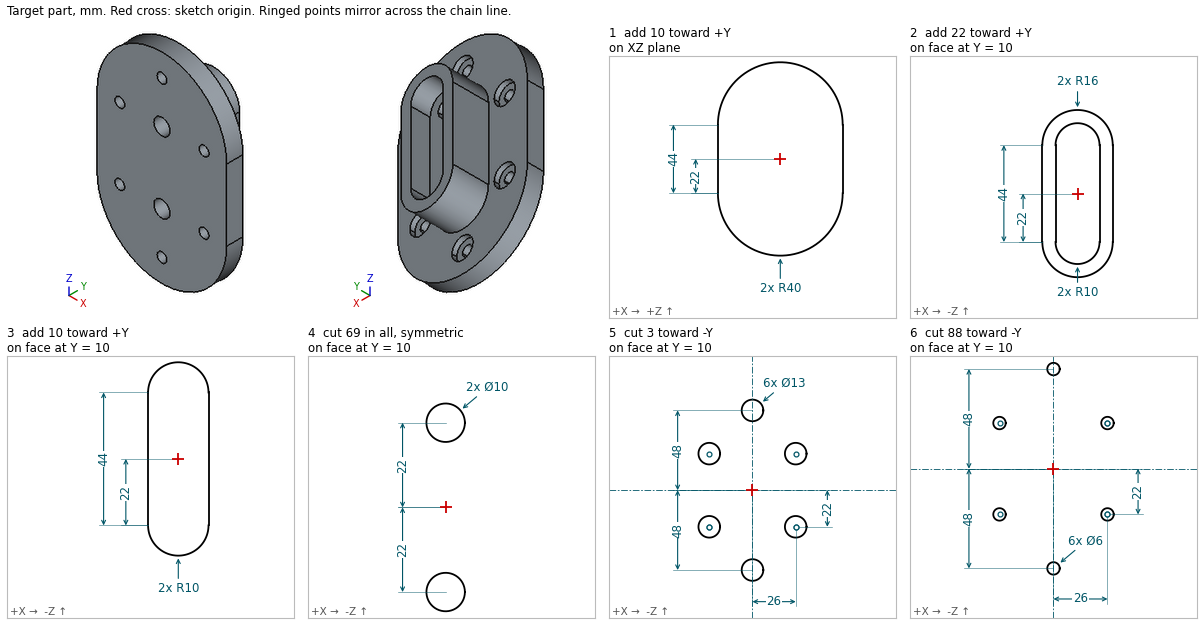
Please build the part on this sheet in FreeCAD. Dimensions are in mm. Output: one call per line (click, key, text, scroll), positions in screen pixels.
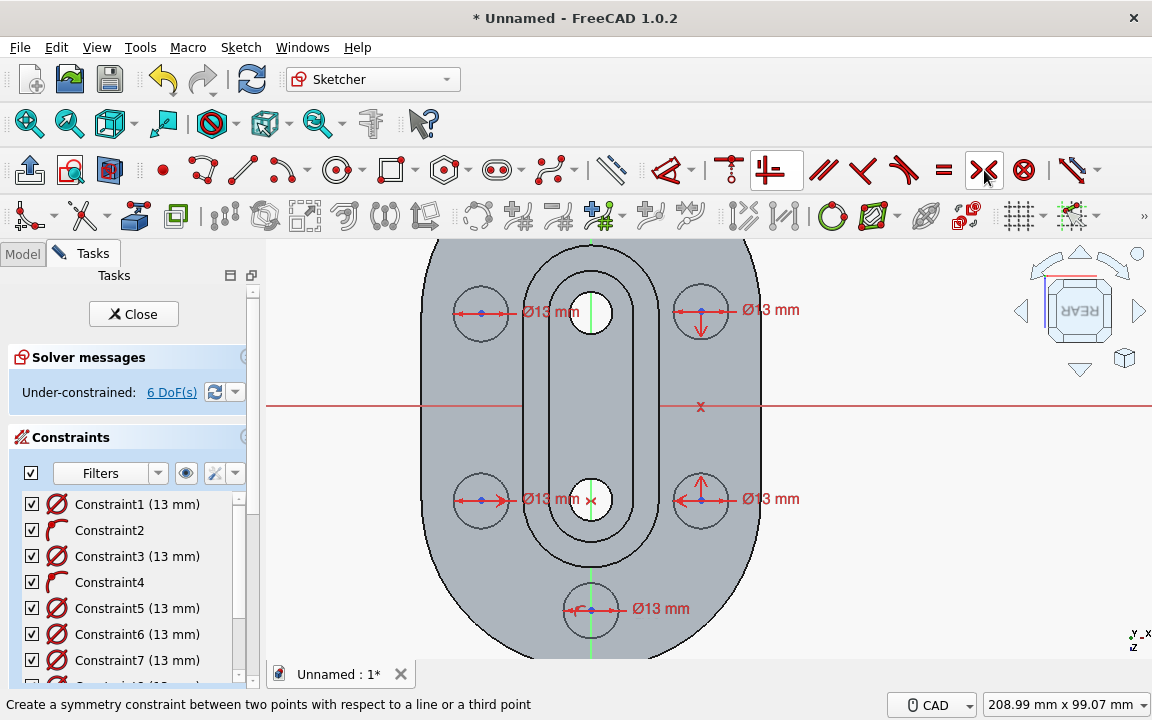
click(481, 501)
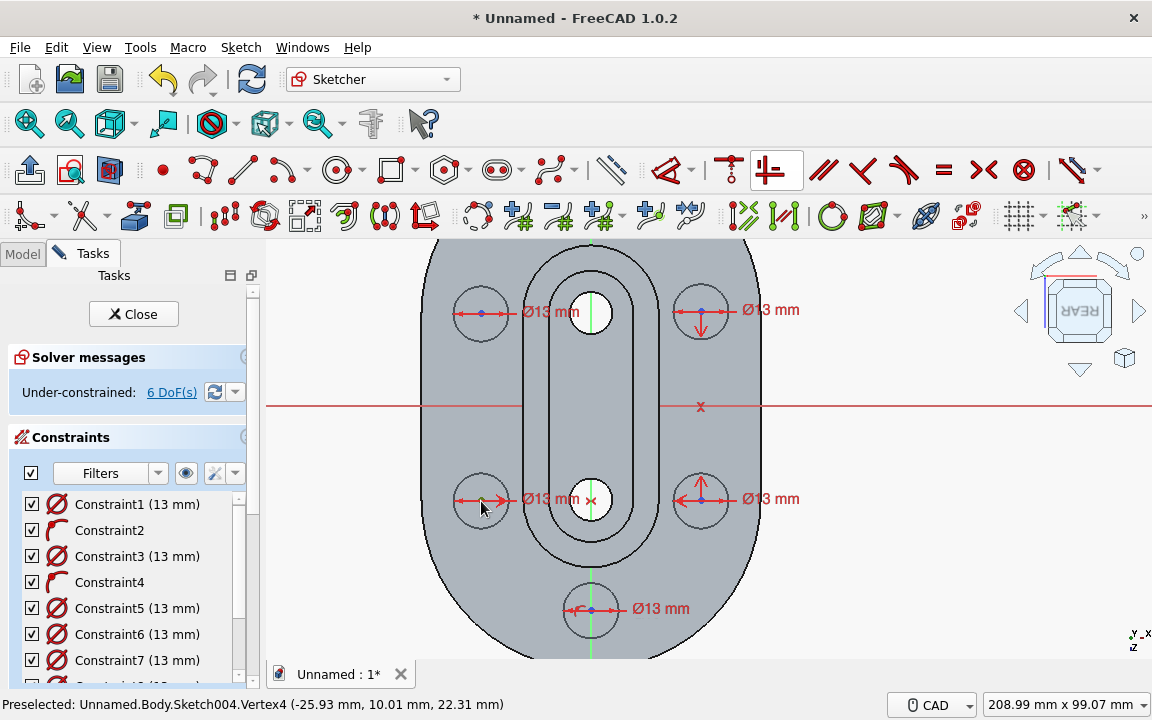
click(481, 314)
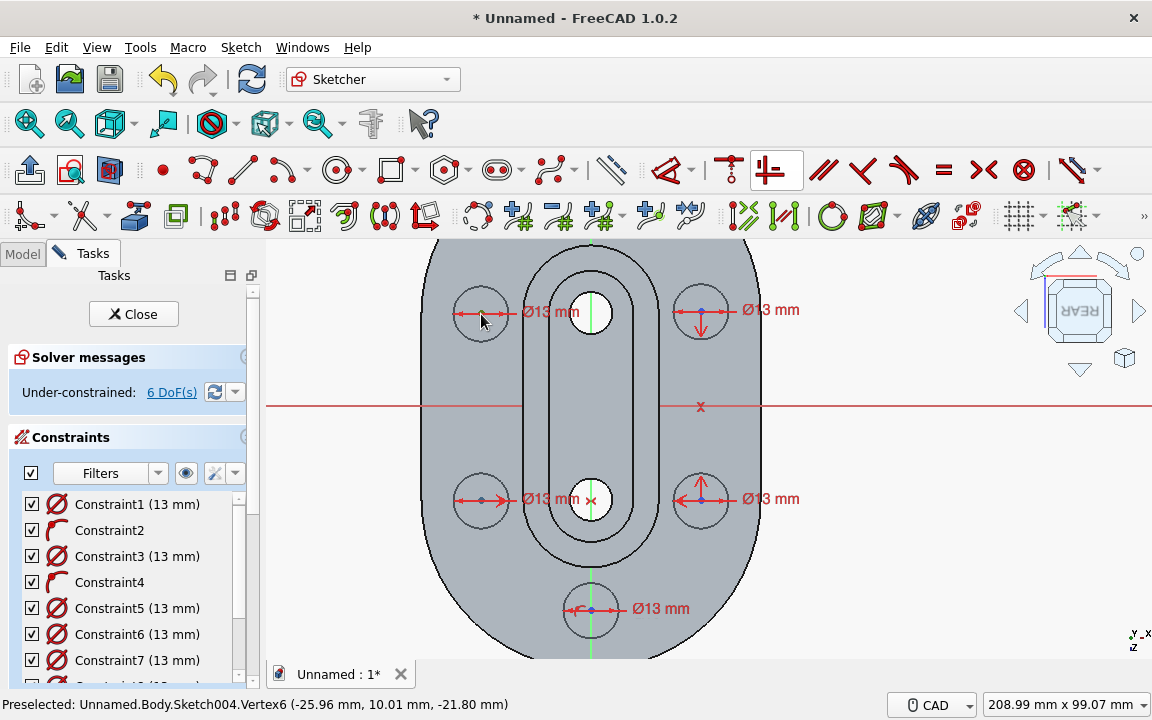
click(344, 406)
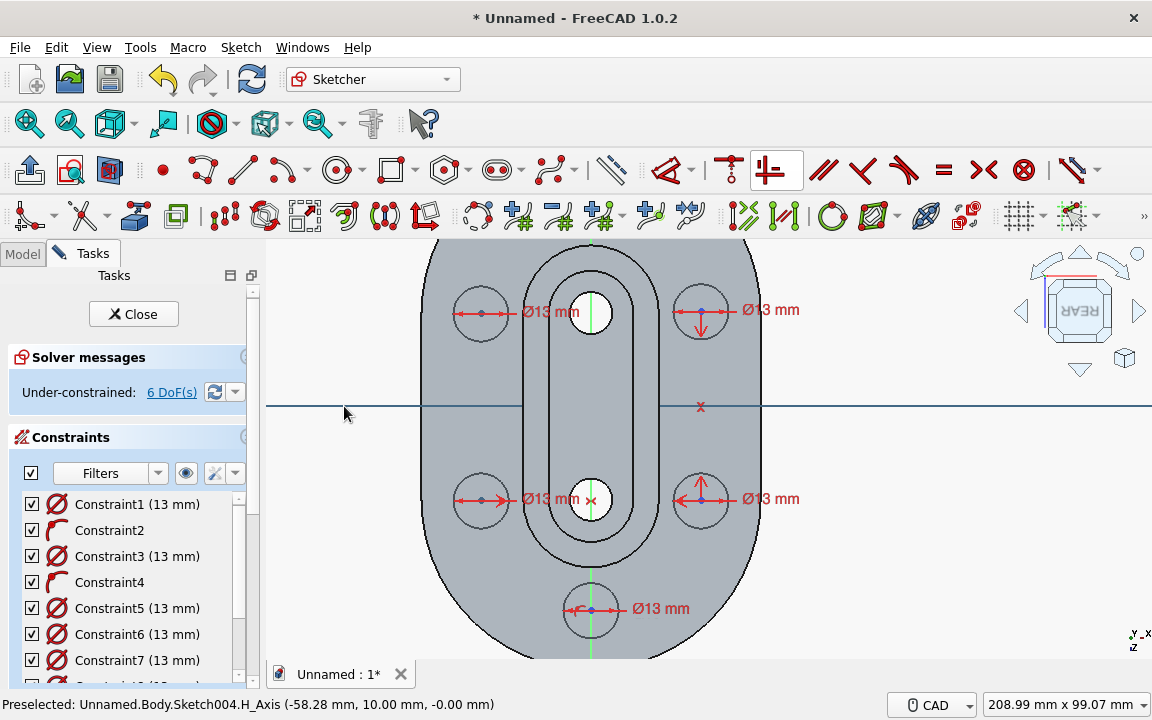
click(984, 170)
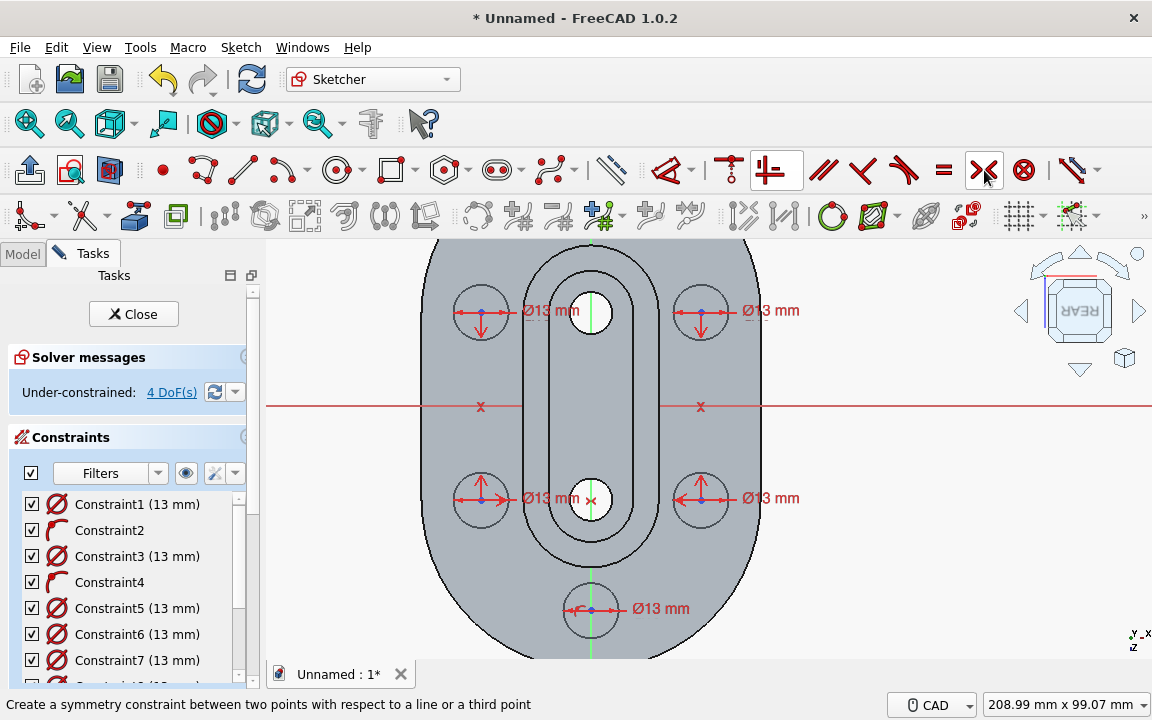
click(666, 170)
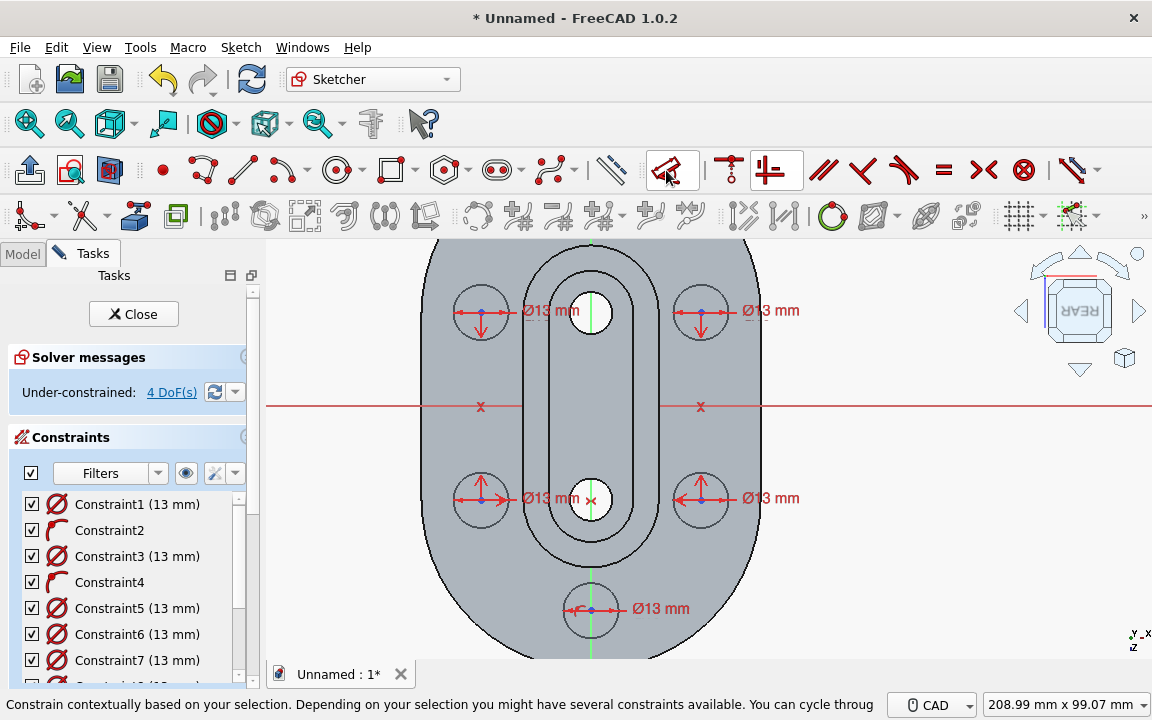
click(591, 611)
click(625, 509)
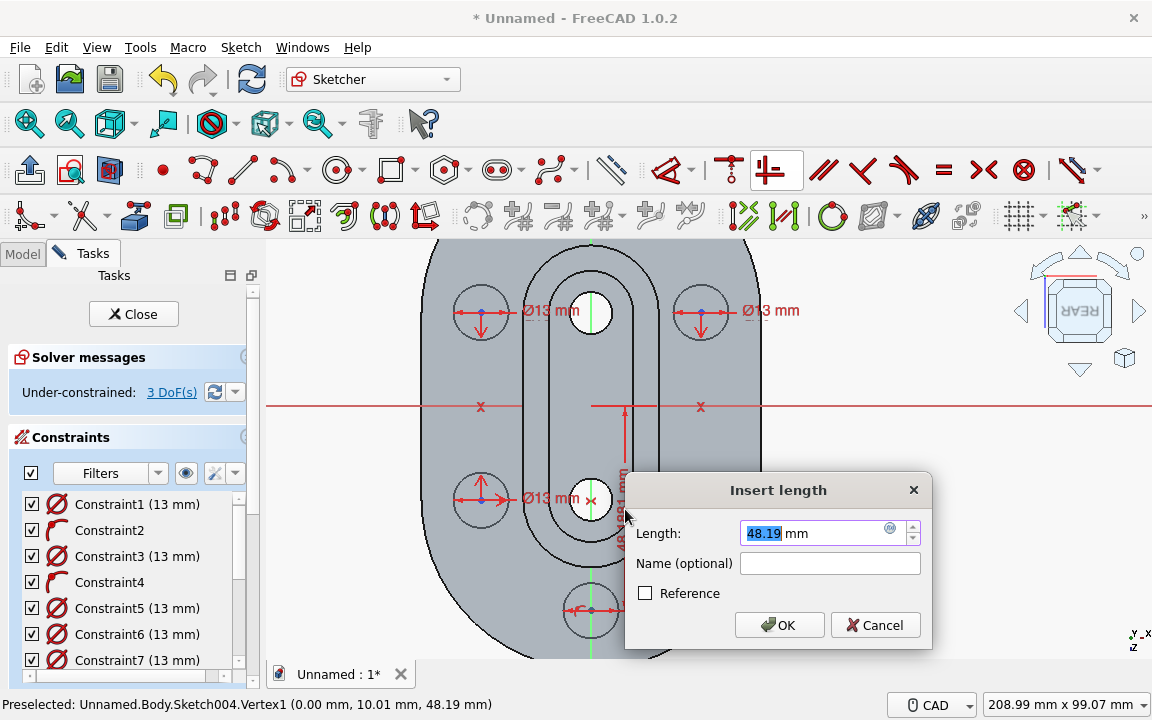
text(48)
key(Return)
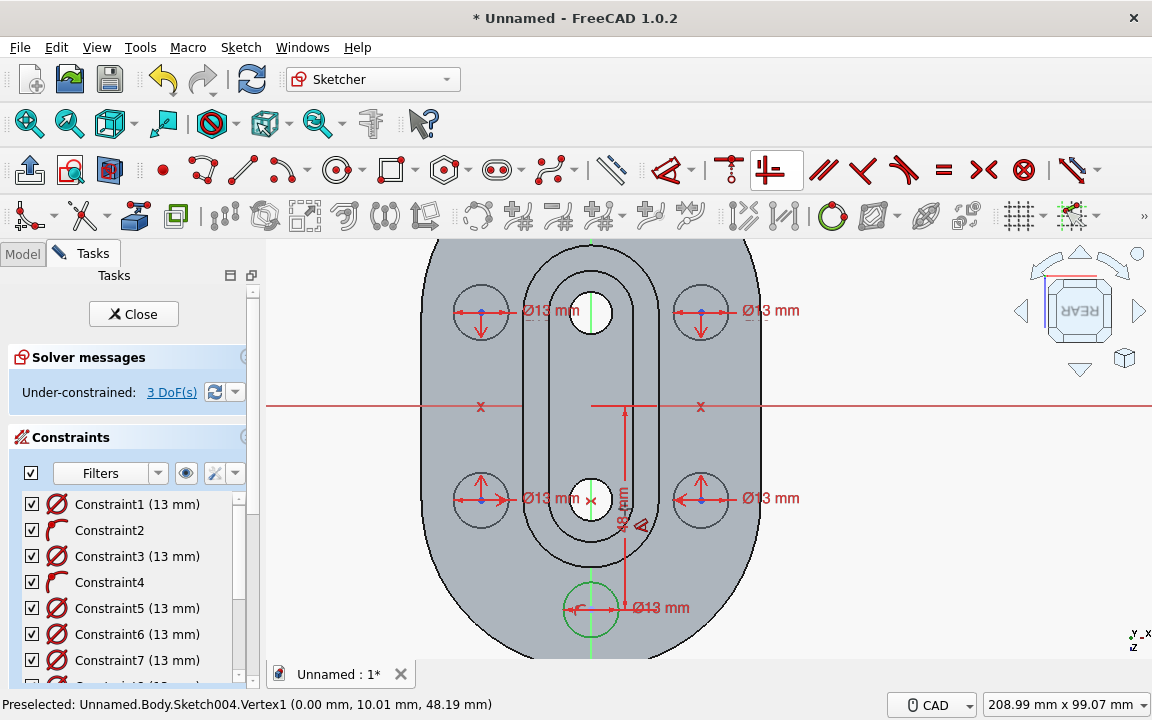
scroll(701, 501, down, 3)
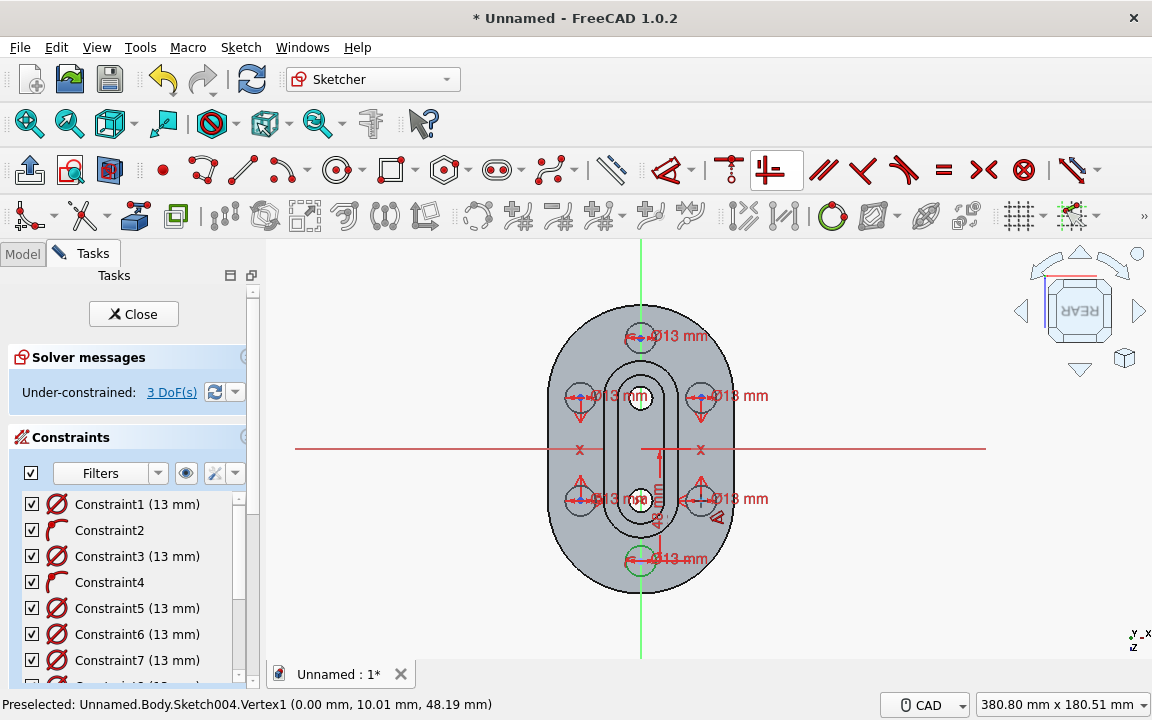
click(641, 338)
click(675, 368)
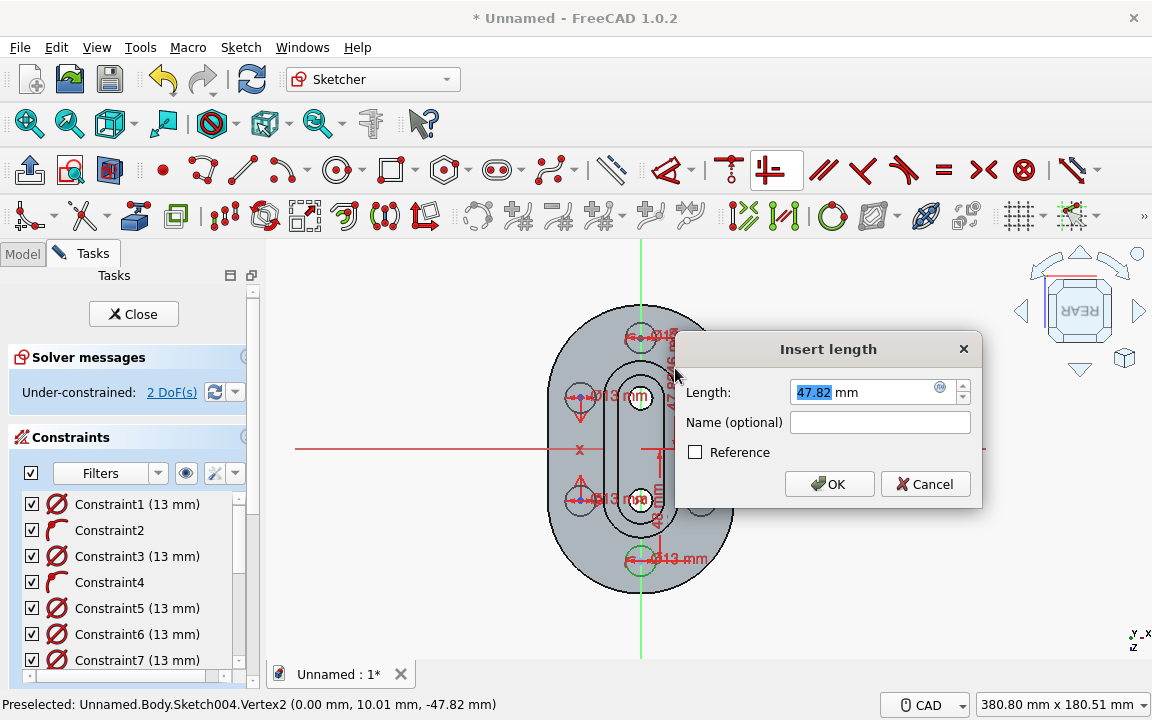
text(48)
key(Return)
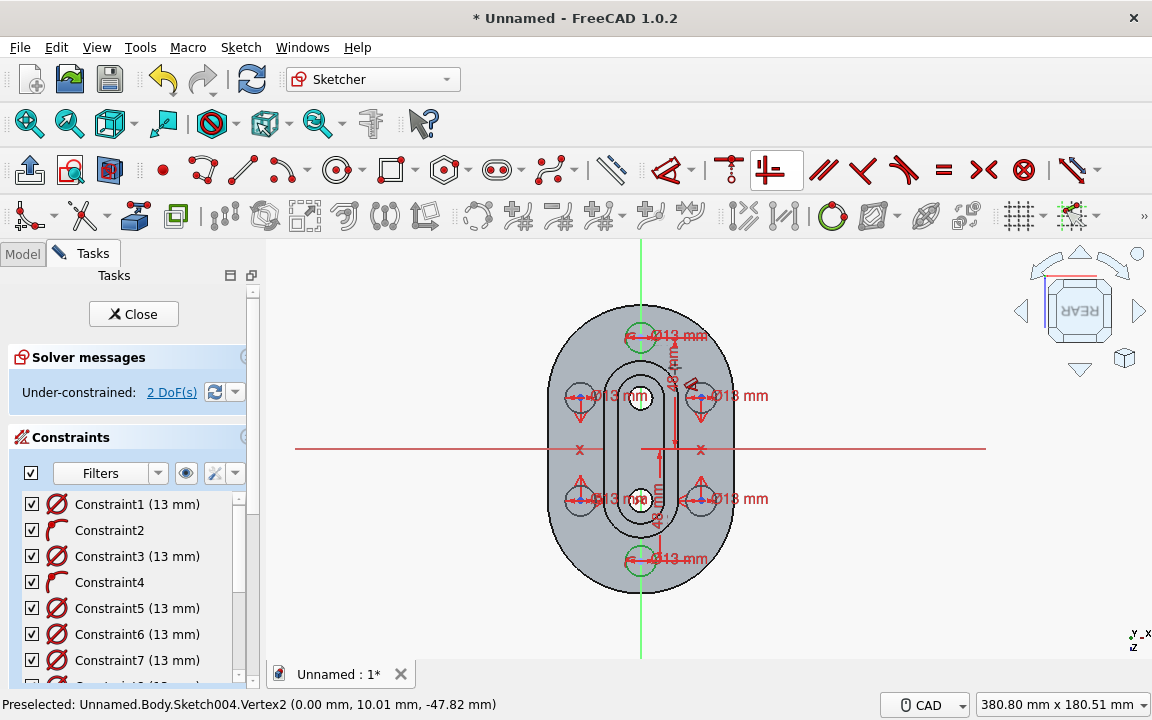
click(701, 501)
click(671, 535)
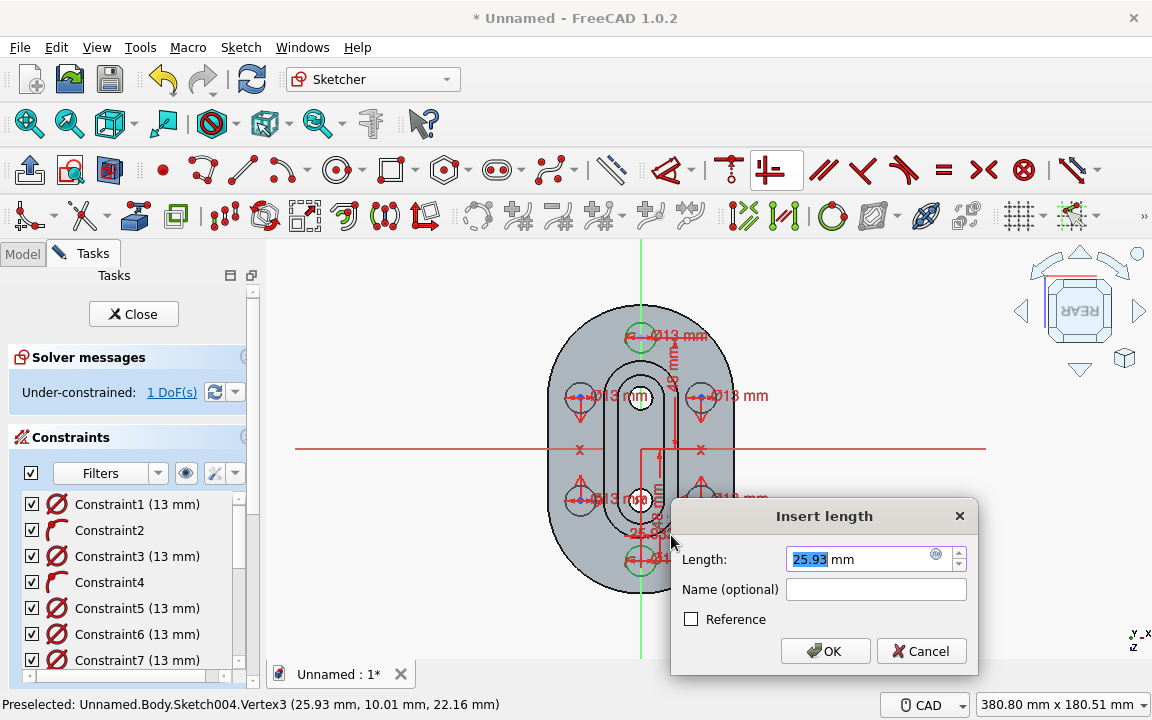
text(26)
key(Return)